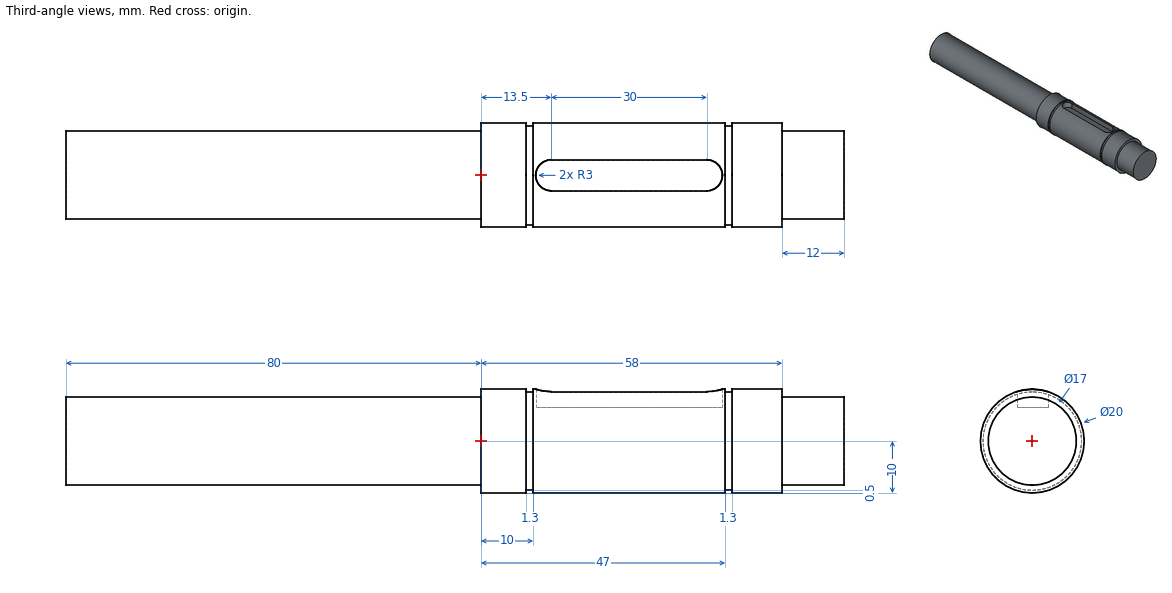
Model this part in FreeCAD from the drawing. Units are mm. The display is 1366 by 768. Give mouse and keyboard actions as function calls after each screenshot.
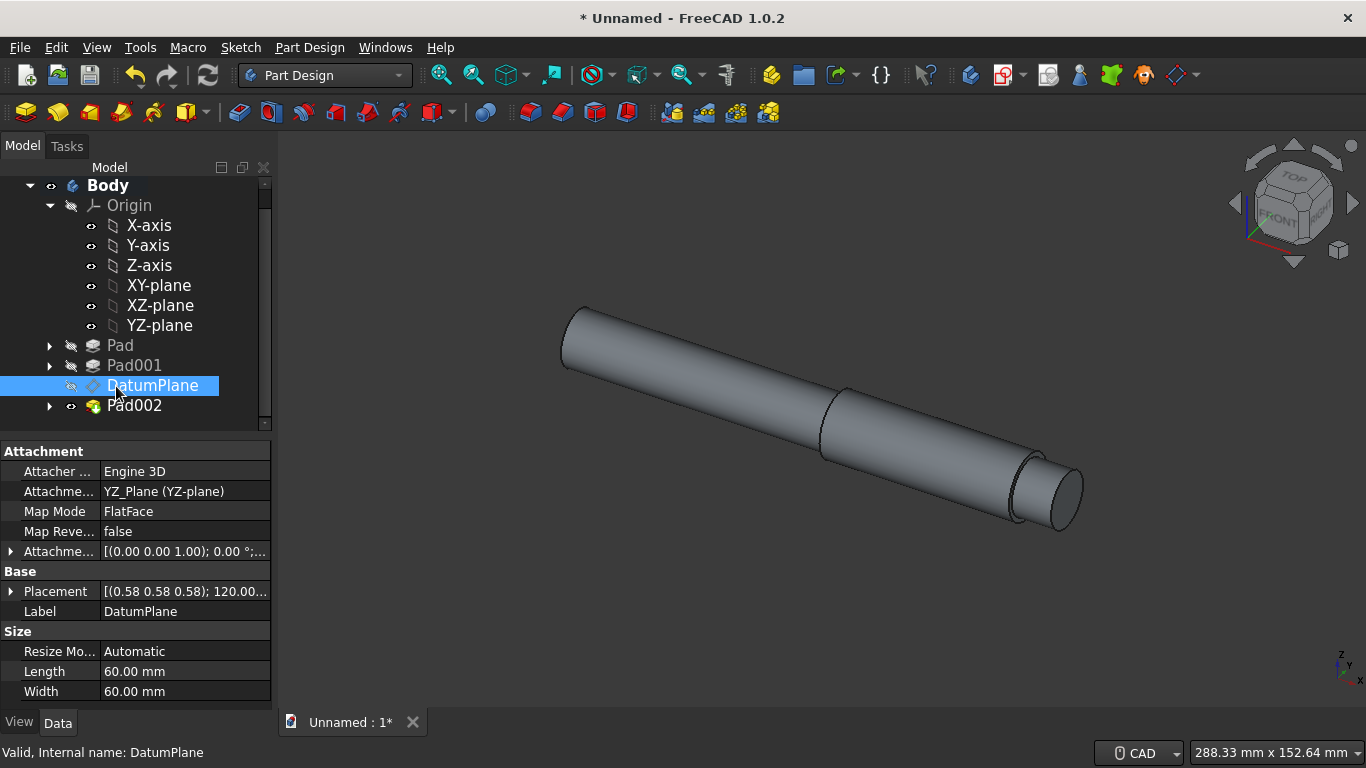
click(136, 286)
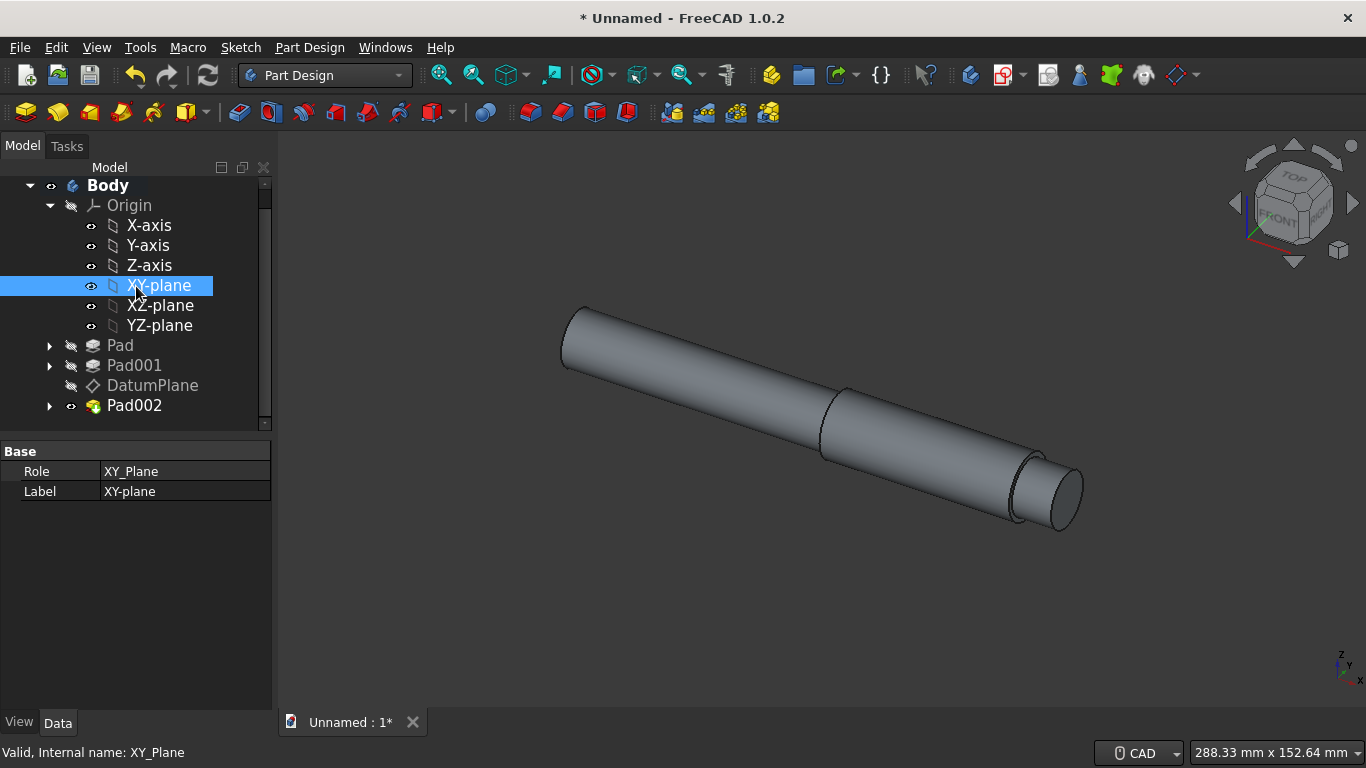
click(1176, 76)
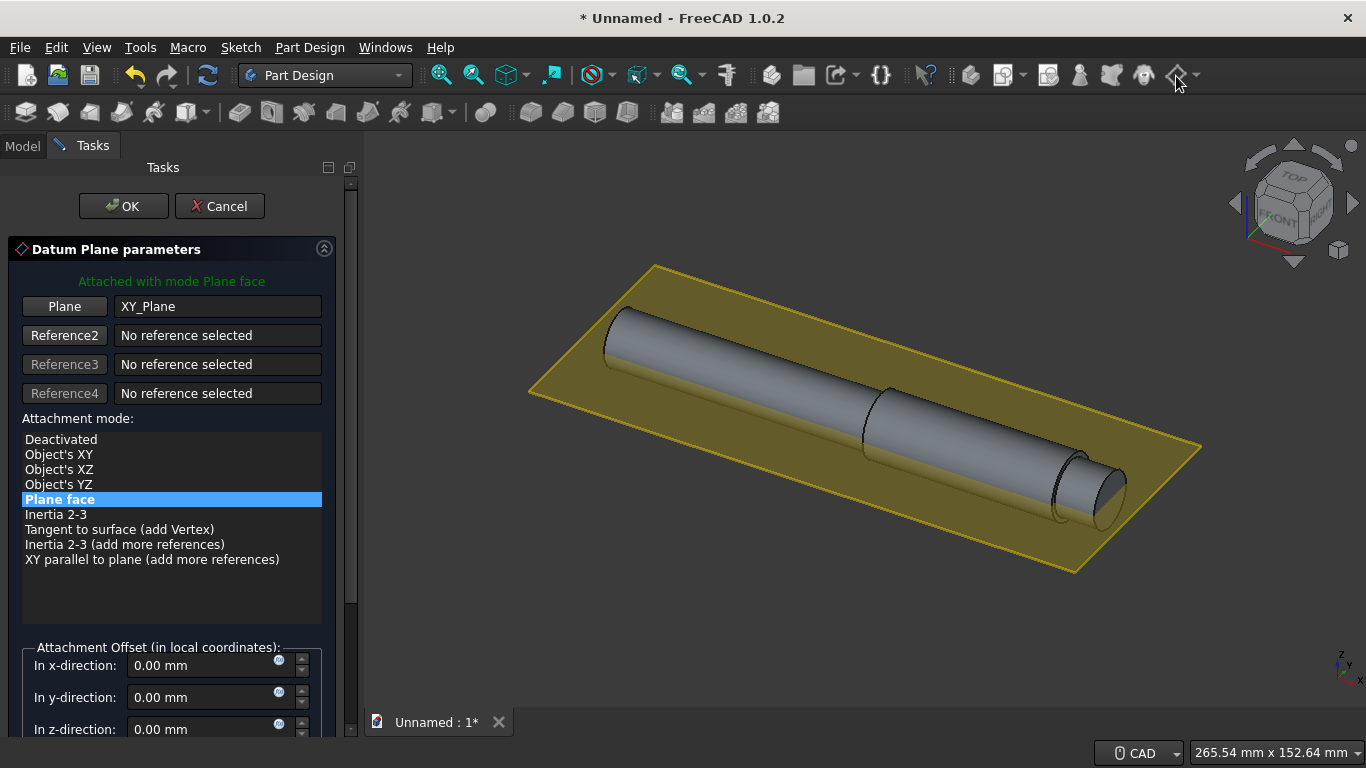
scroll(351, 456, down, 2)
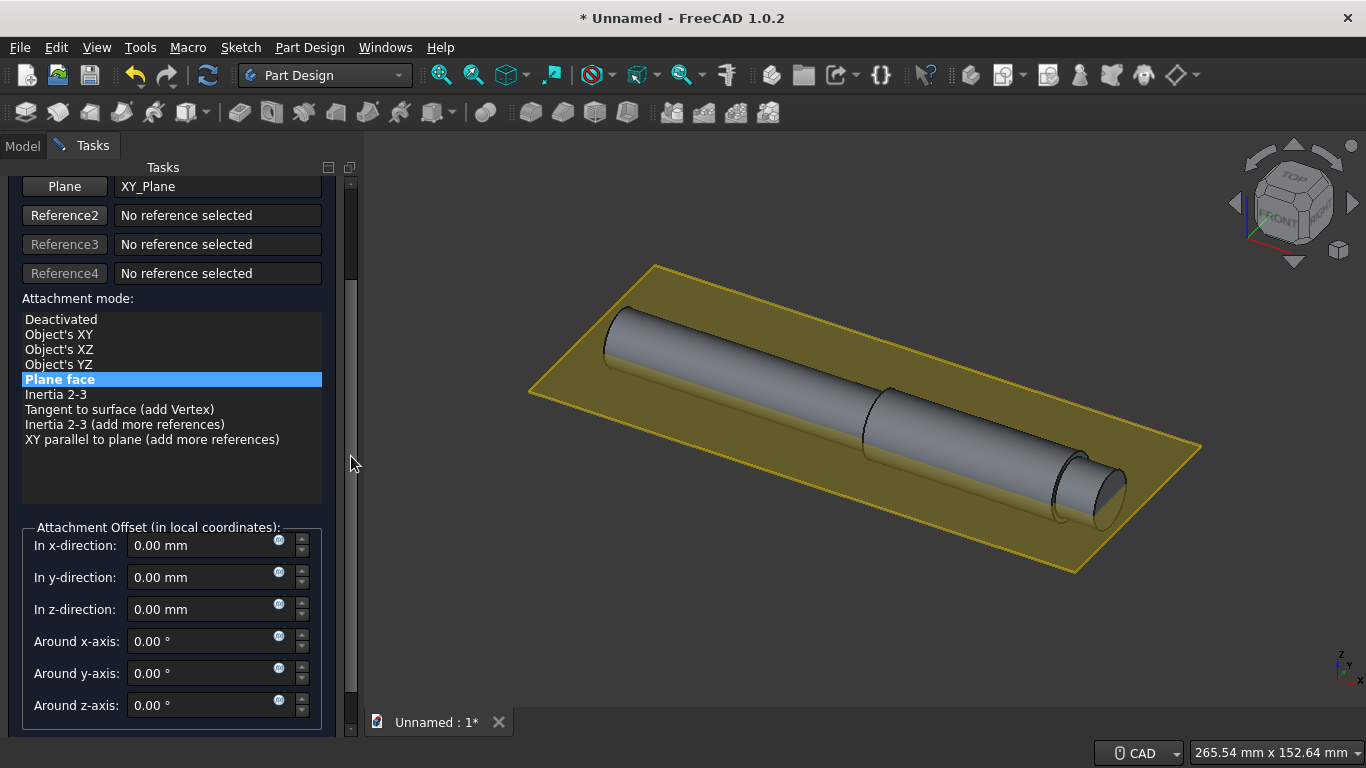
triple_click(210, 609)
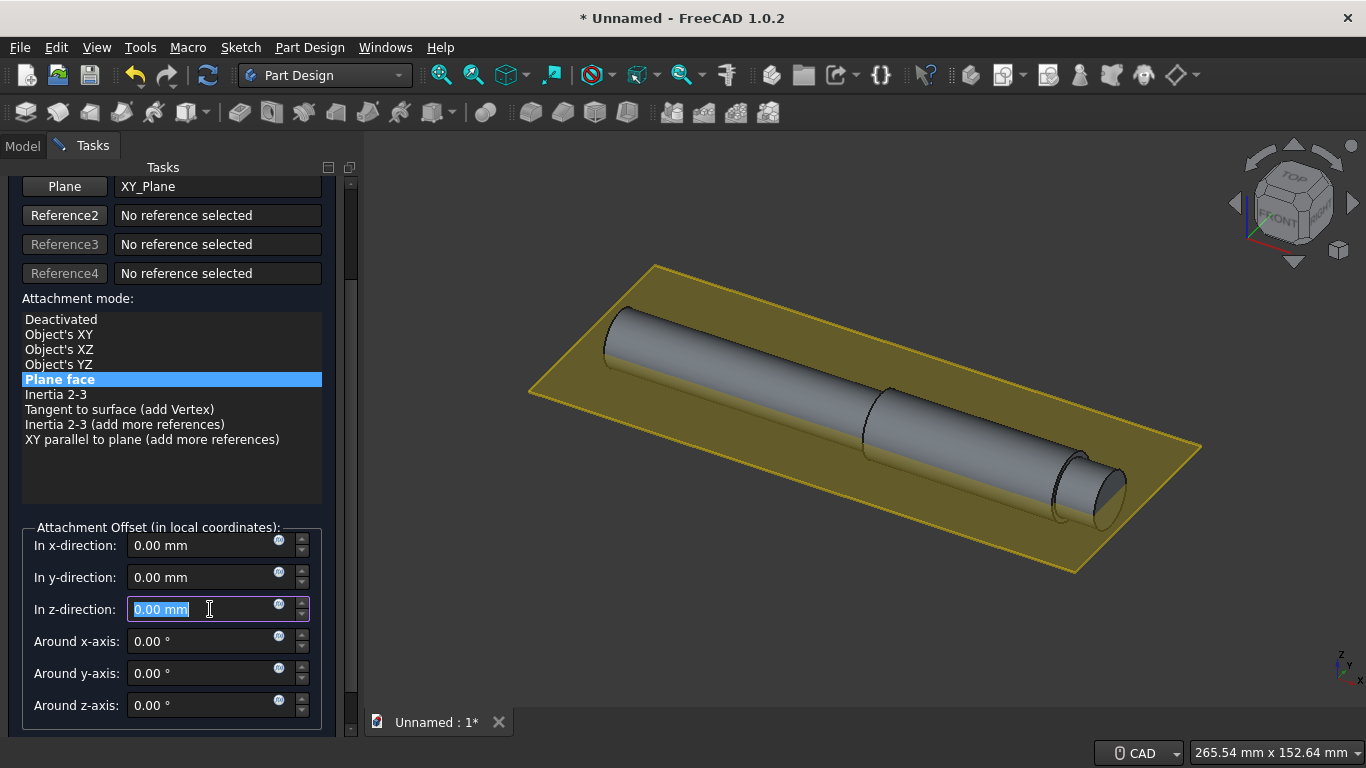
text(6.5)
key(Tab)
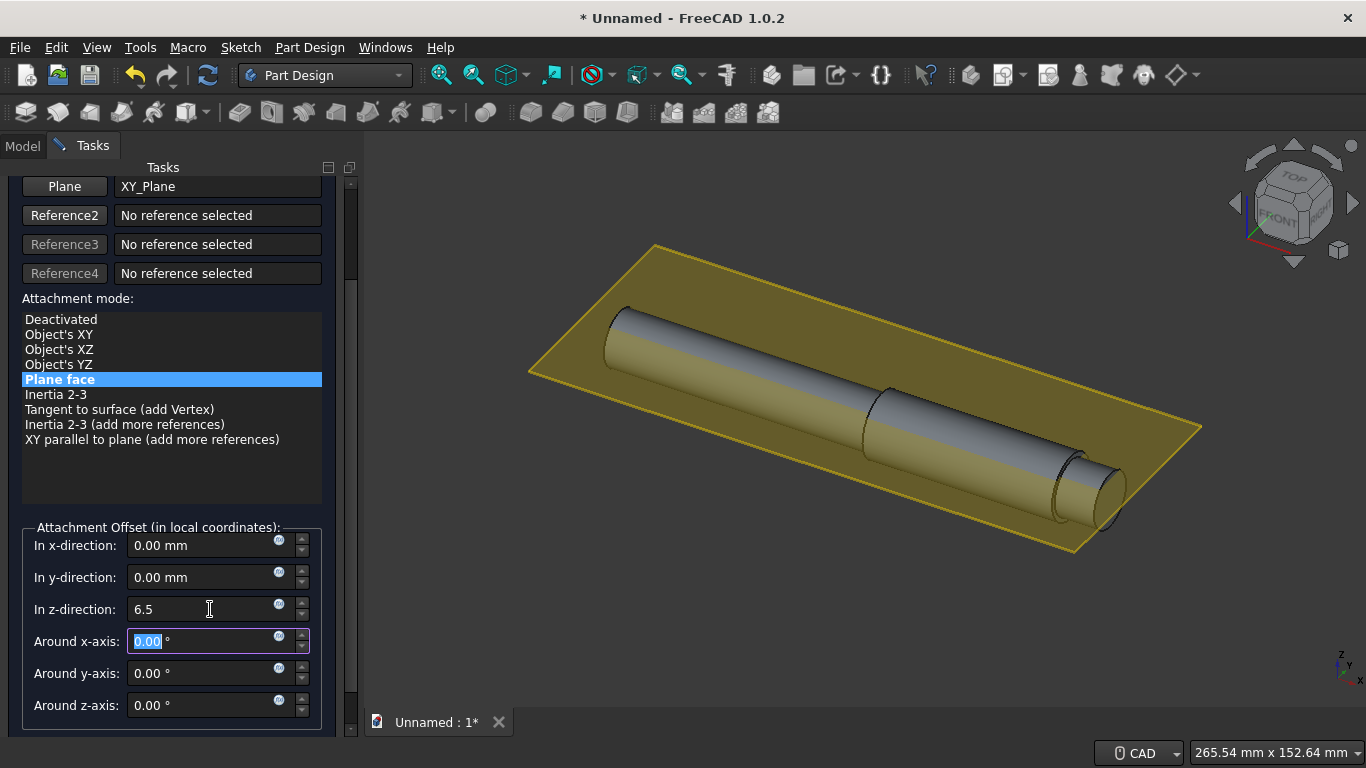
scroll(351, 456, up, 3)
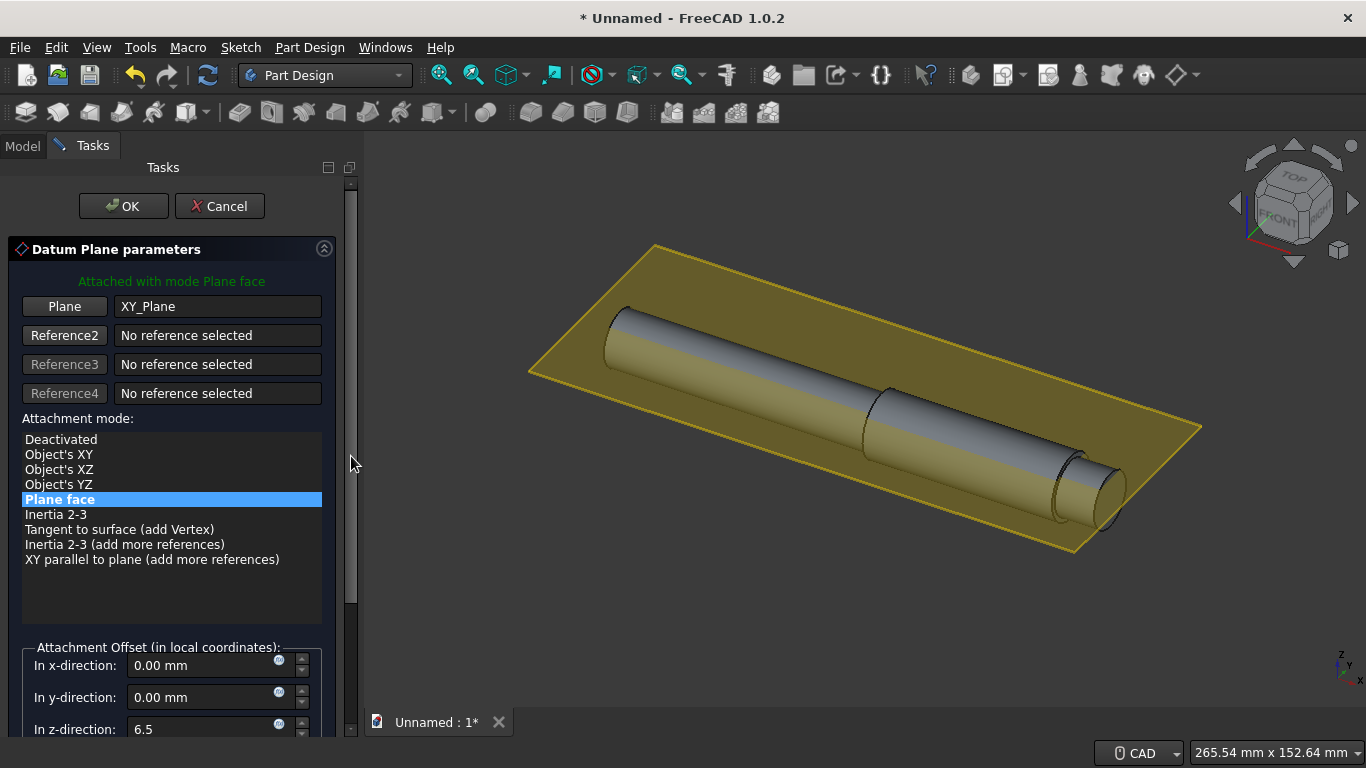
click(124, 206)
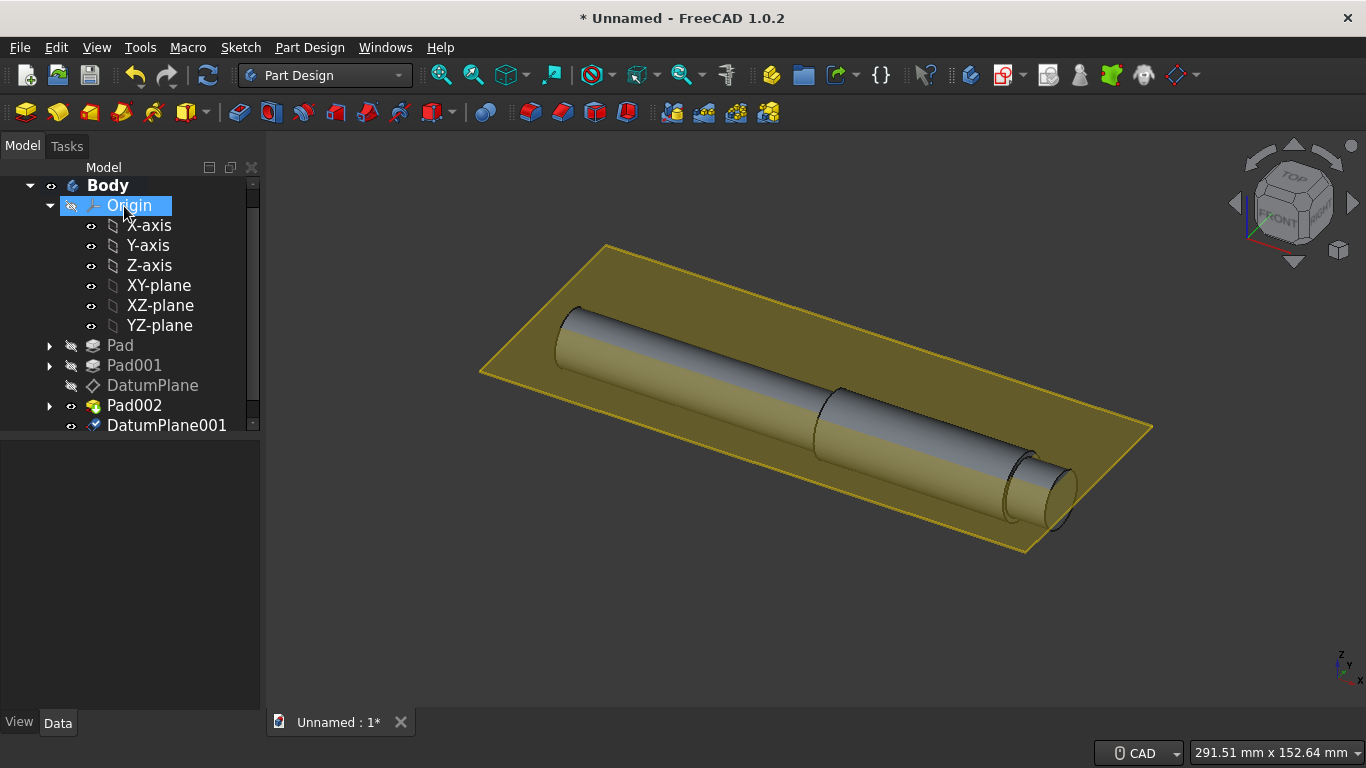
click(116, 426)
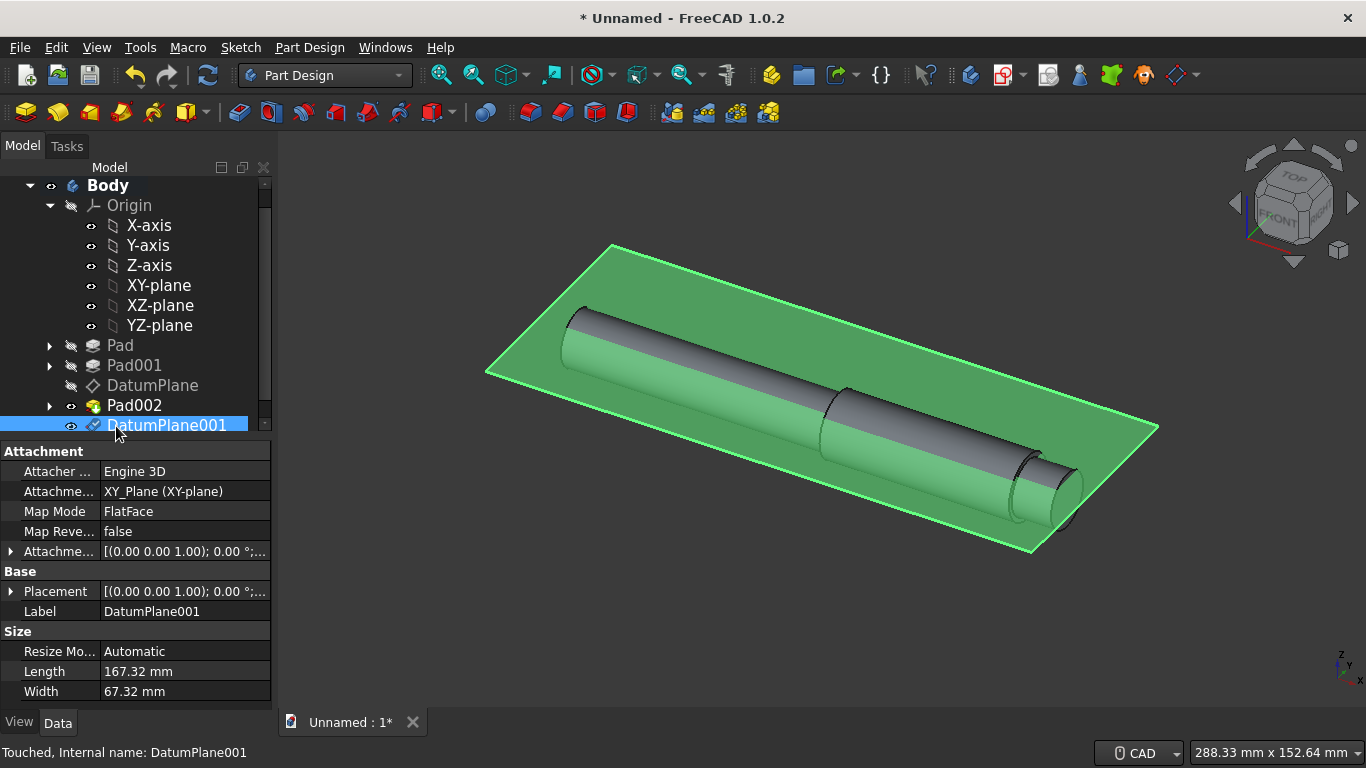
click(1004, 76)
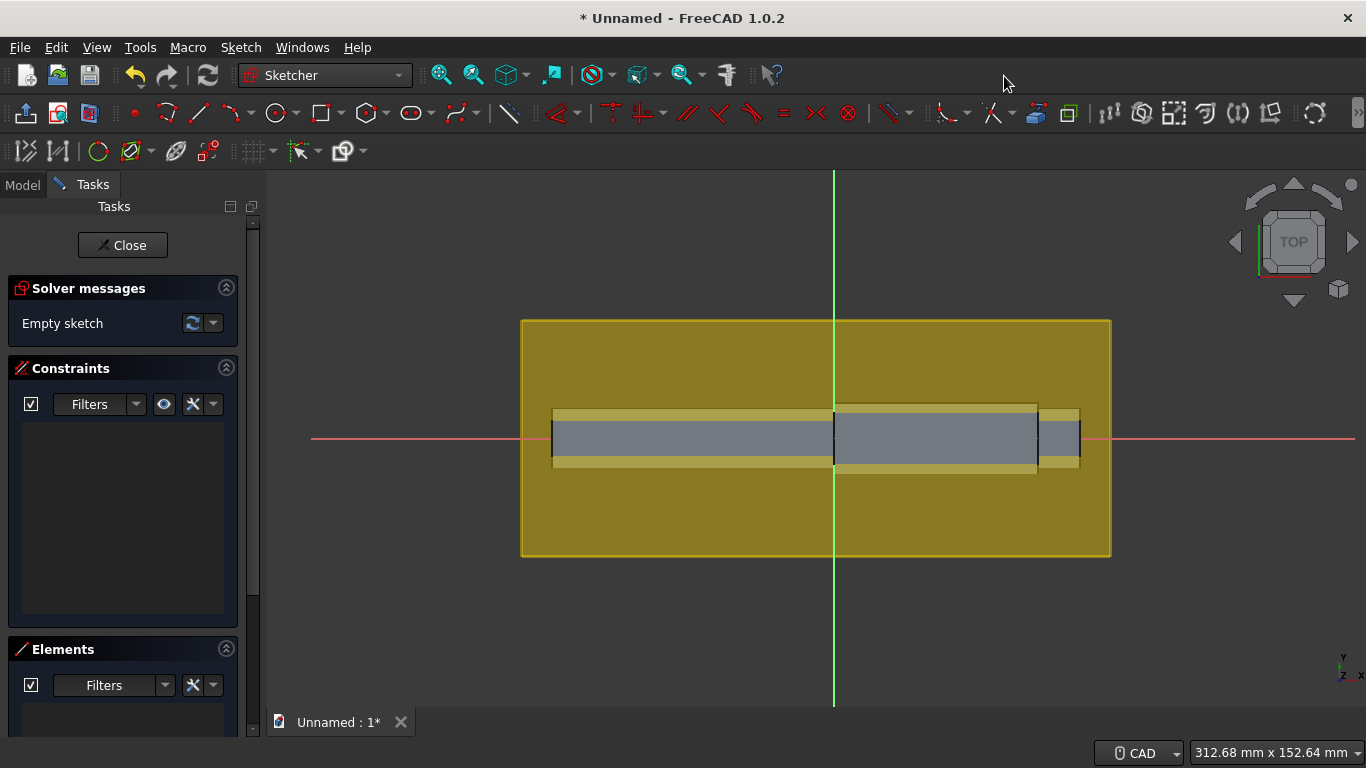
key(q)
key(s)